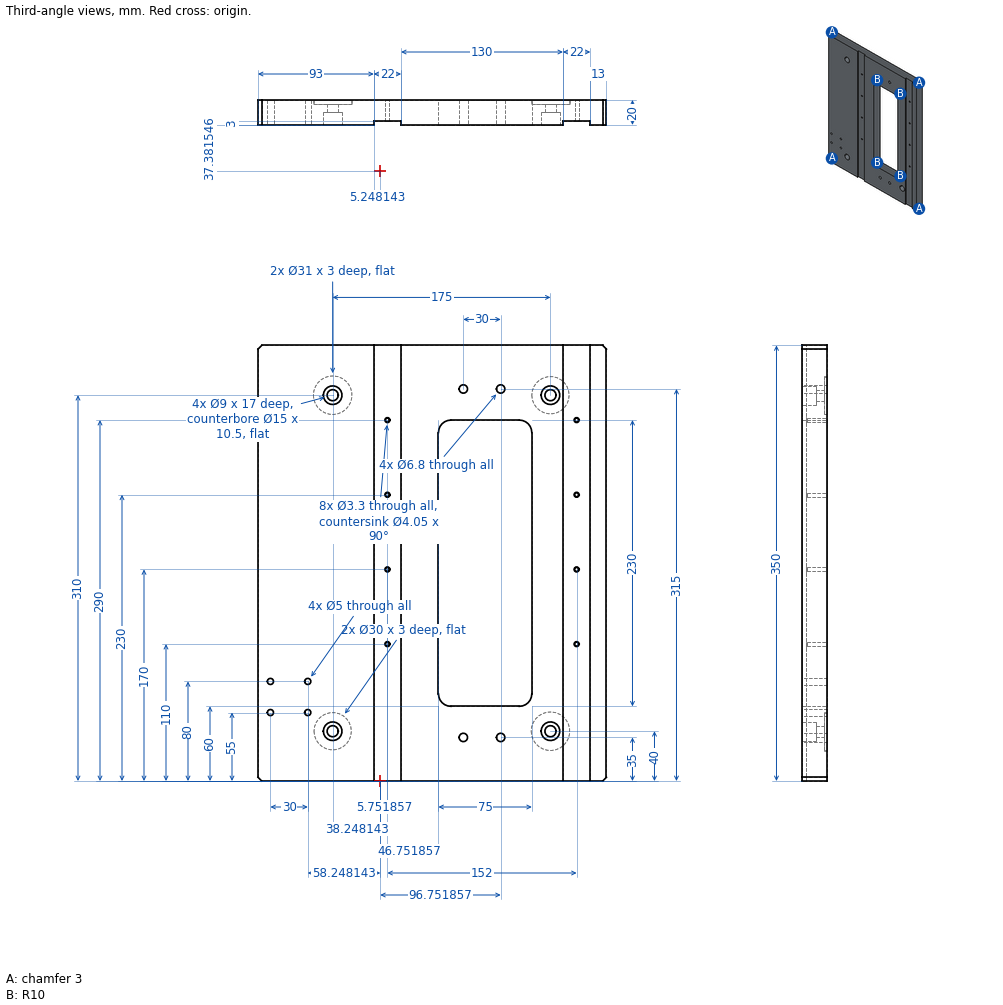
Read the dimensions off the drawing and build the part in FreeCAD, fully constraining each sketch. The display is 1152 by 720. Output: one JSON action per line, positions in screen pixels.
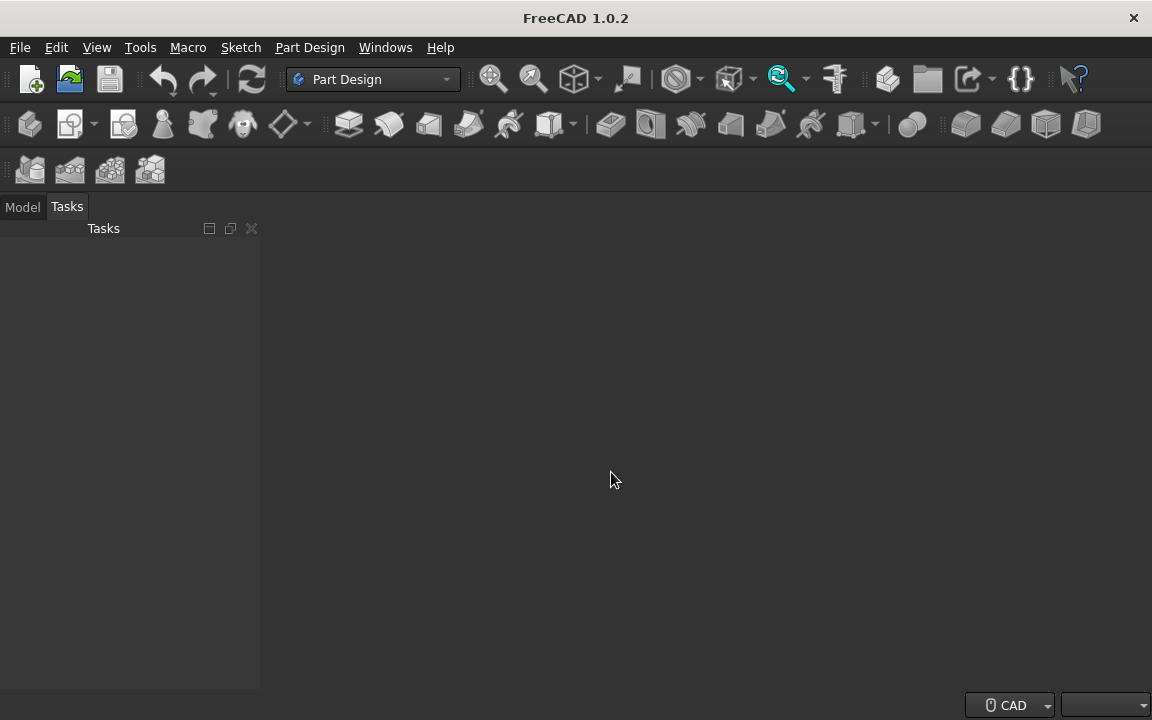
{"action": "left_click", "coordinate": [30, 80]}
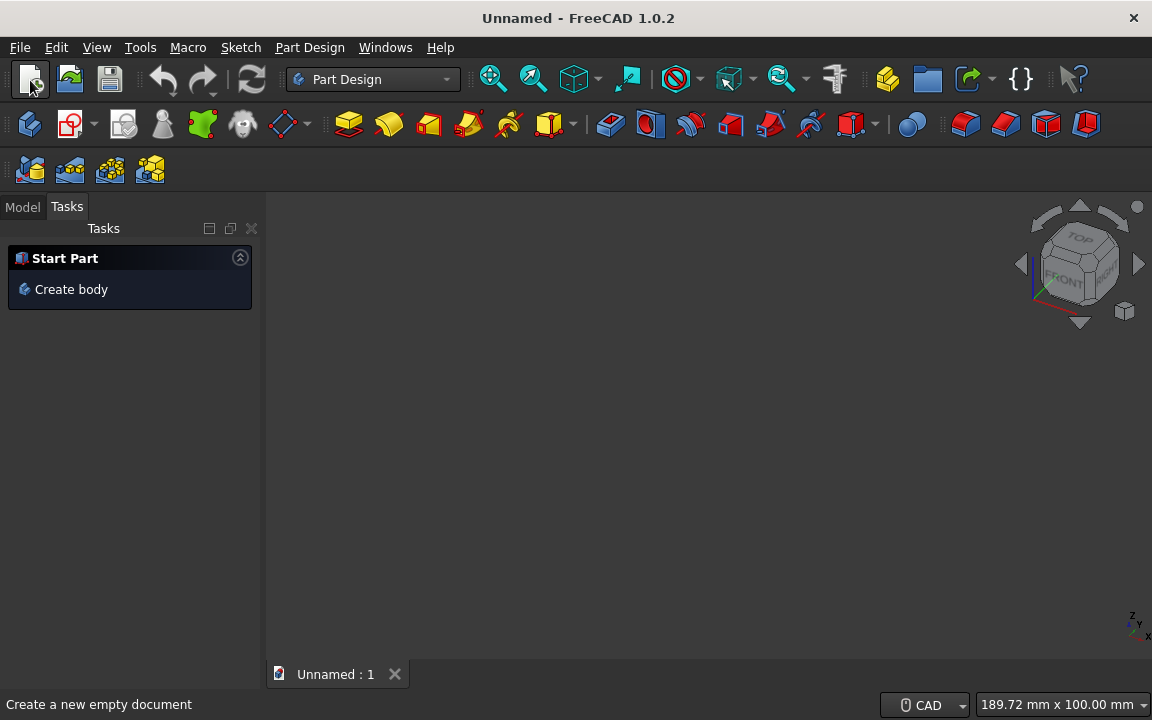
{"action": "left_click", "coordinate": [70, 124]}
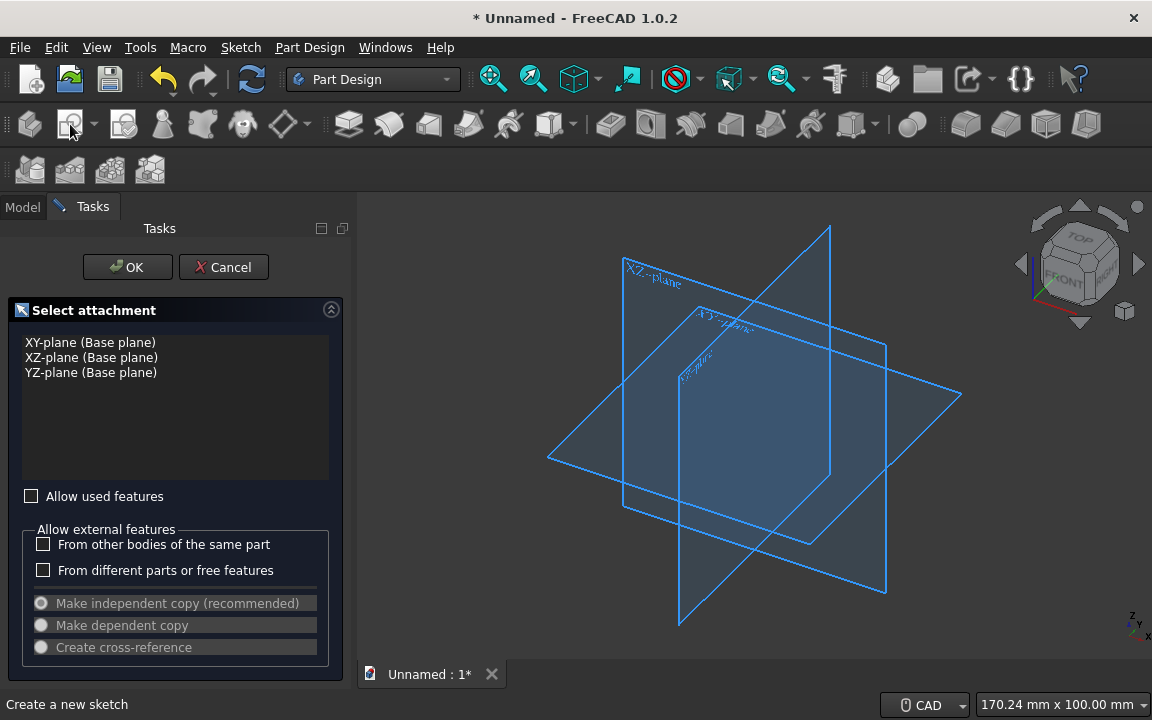
{"action": "left_click", "coordinate": [82, 342]}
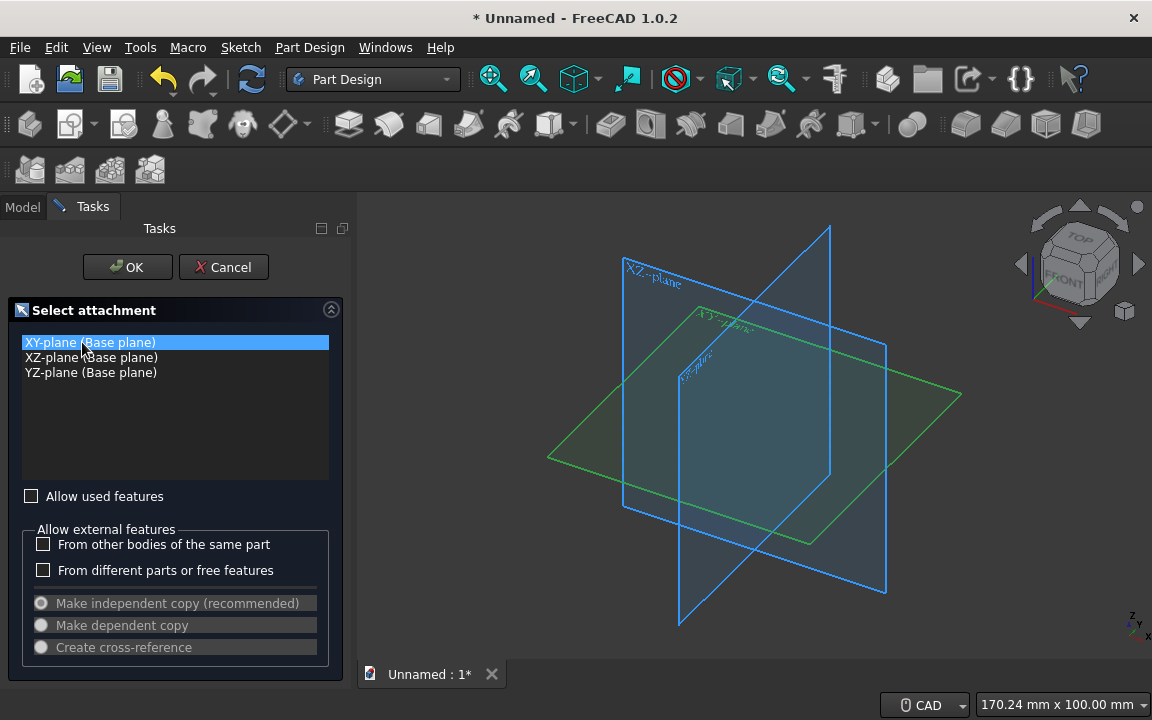
{"action": "left_click", "coordinate": [128, 267]}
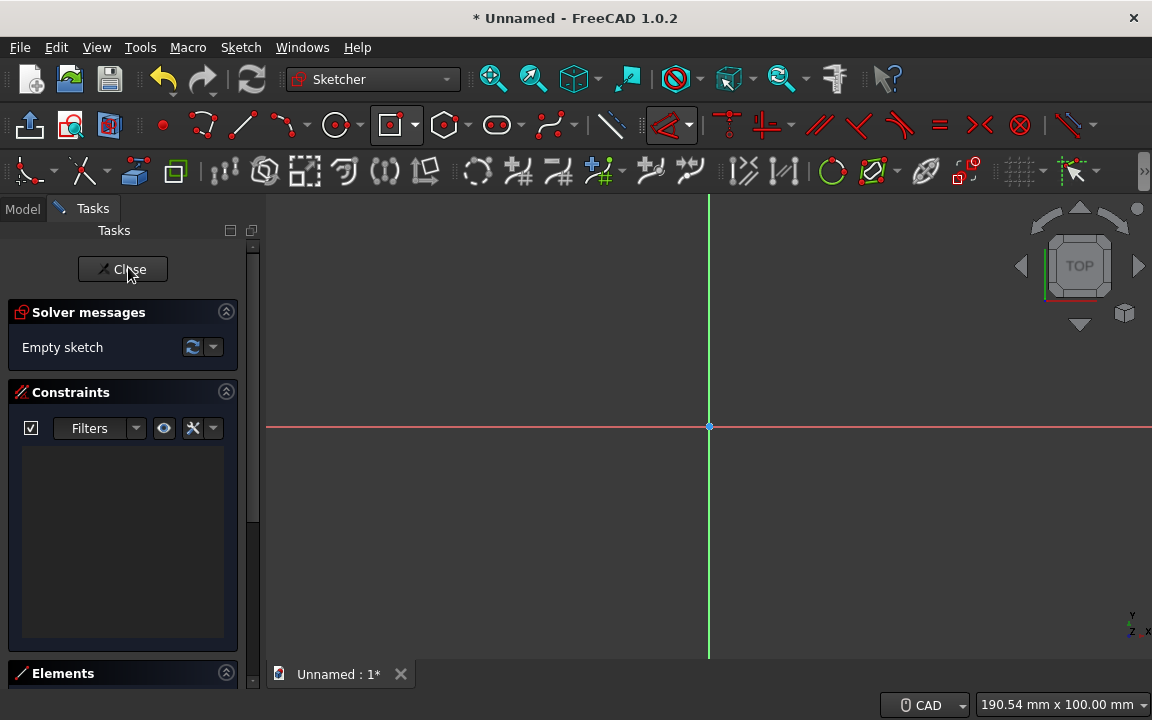
{"action": "scroll", "coordinate": [488, 504], "scroll_direction": "down", "scroll_amount": 5}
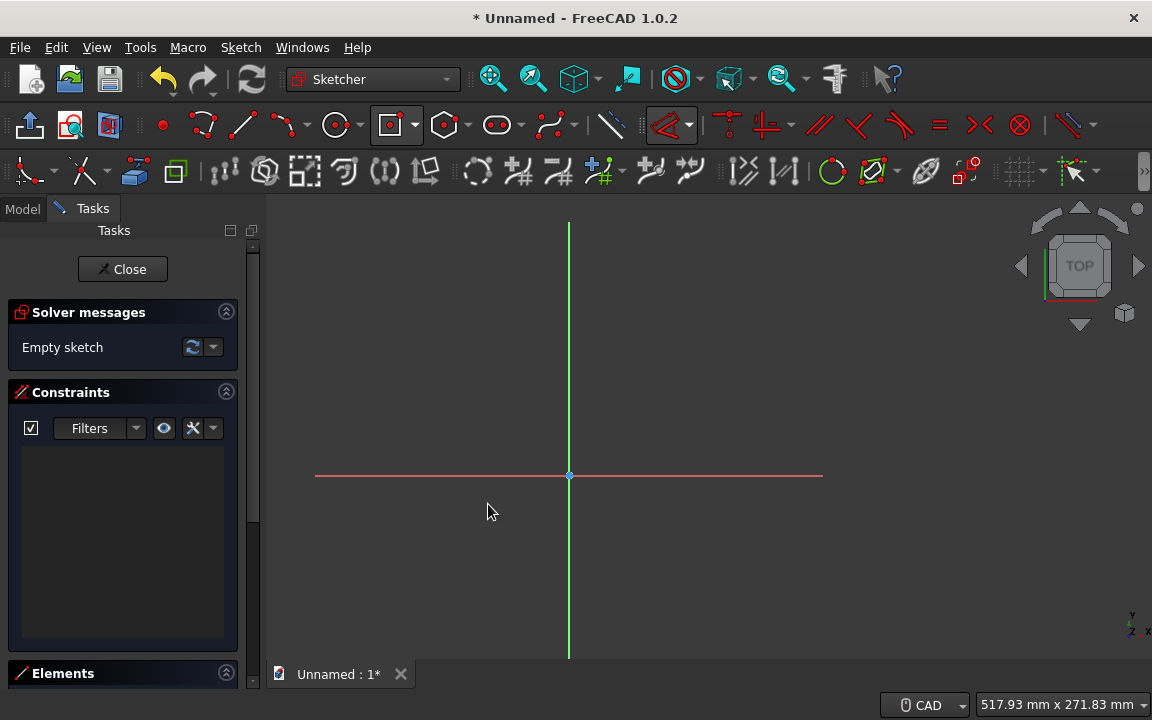
{"action": "left_click", "coordinate": [204, 126]}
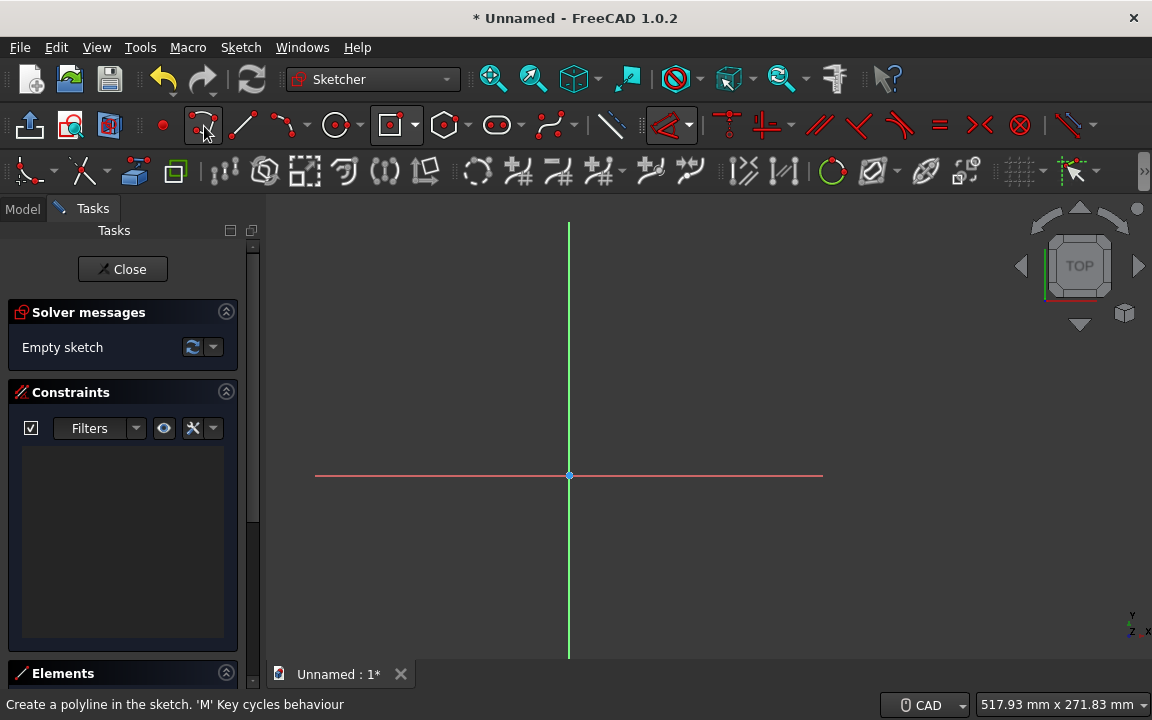
{"action": "scroll", "coordinate": [560, 412], "scroll_direction": "up", "scroll_amount": 3}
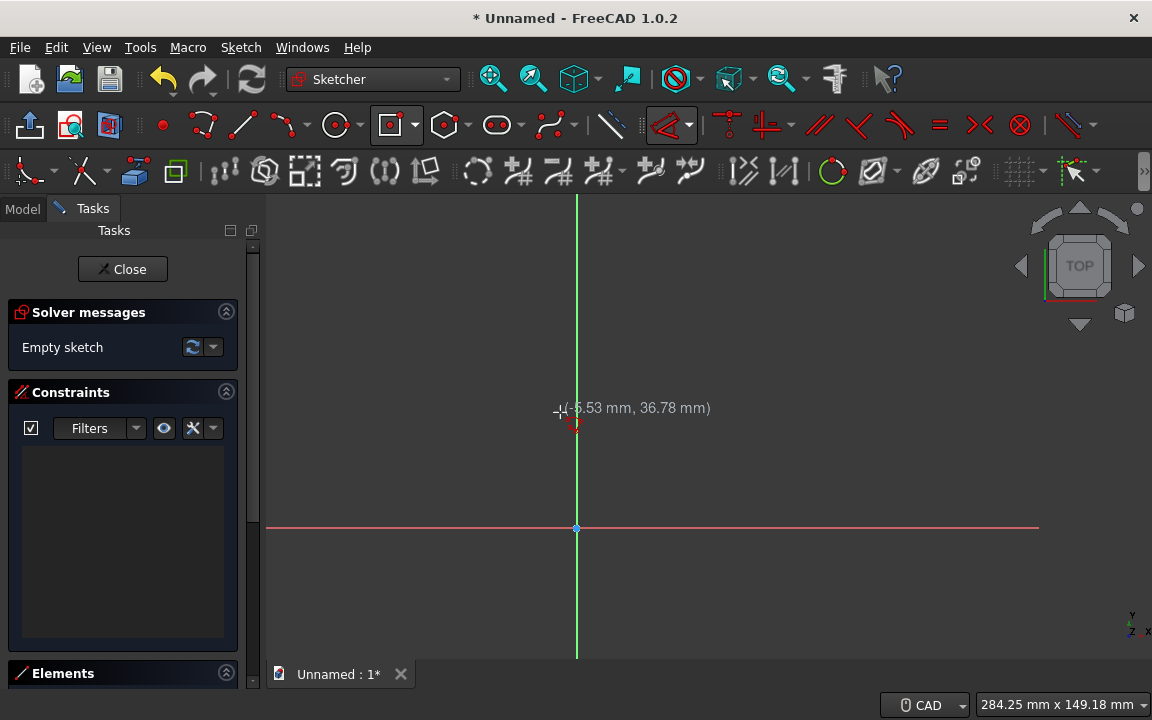
{"action": "left_click", "coordinate": [561, 412]}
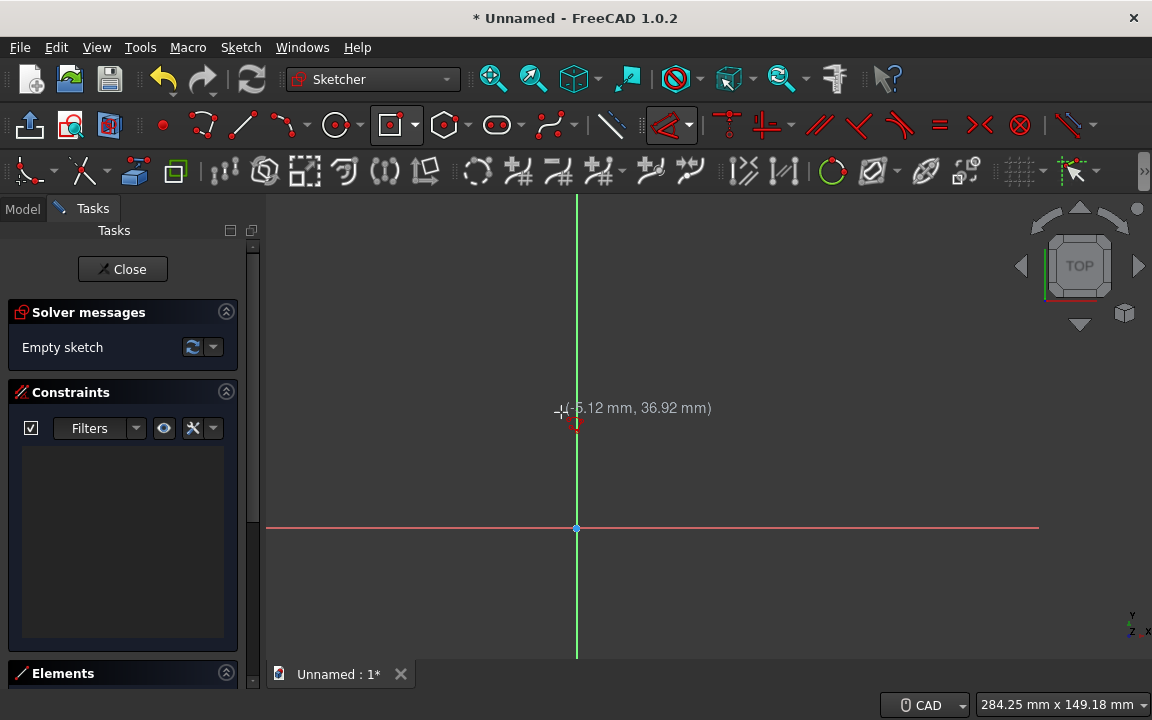
{"action": "scroll", "coordinate": [561, 402], "scroll_direction": "up", "scroll_amount": 3}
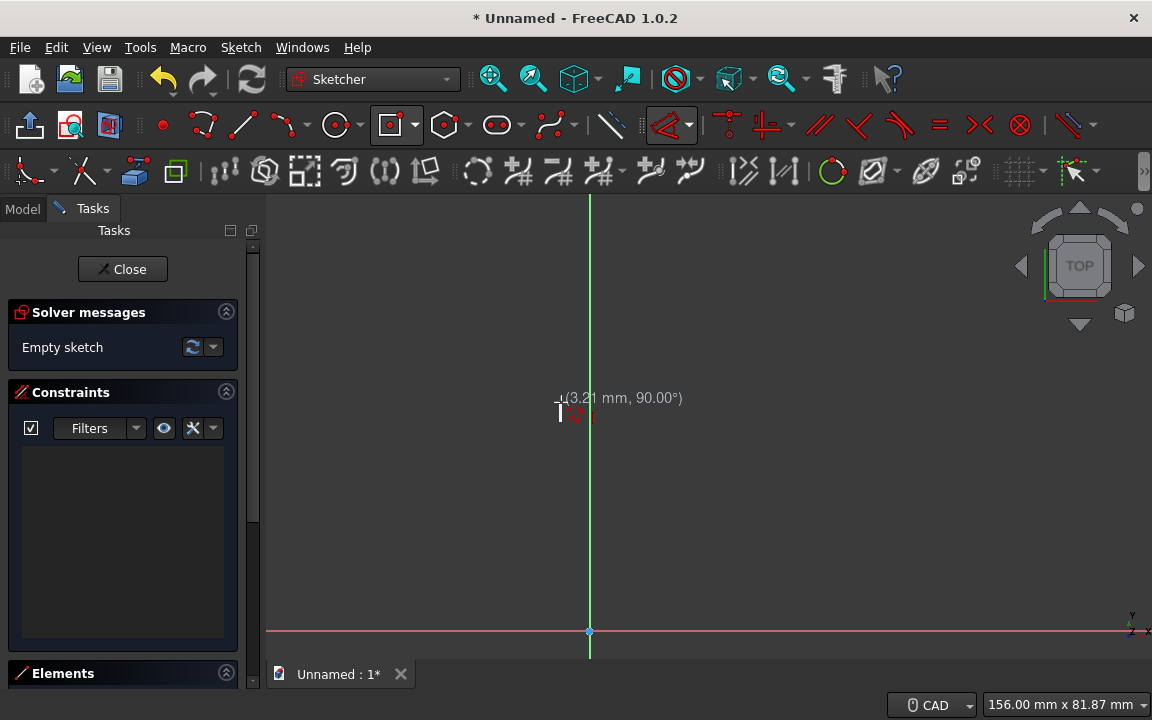
{"action": "left_click", "coordinate": [561, 402]}
{"action": "left_click", "coordinate": [685, 402]}
{"action": "left_click", "coordinate": [685, 419]}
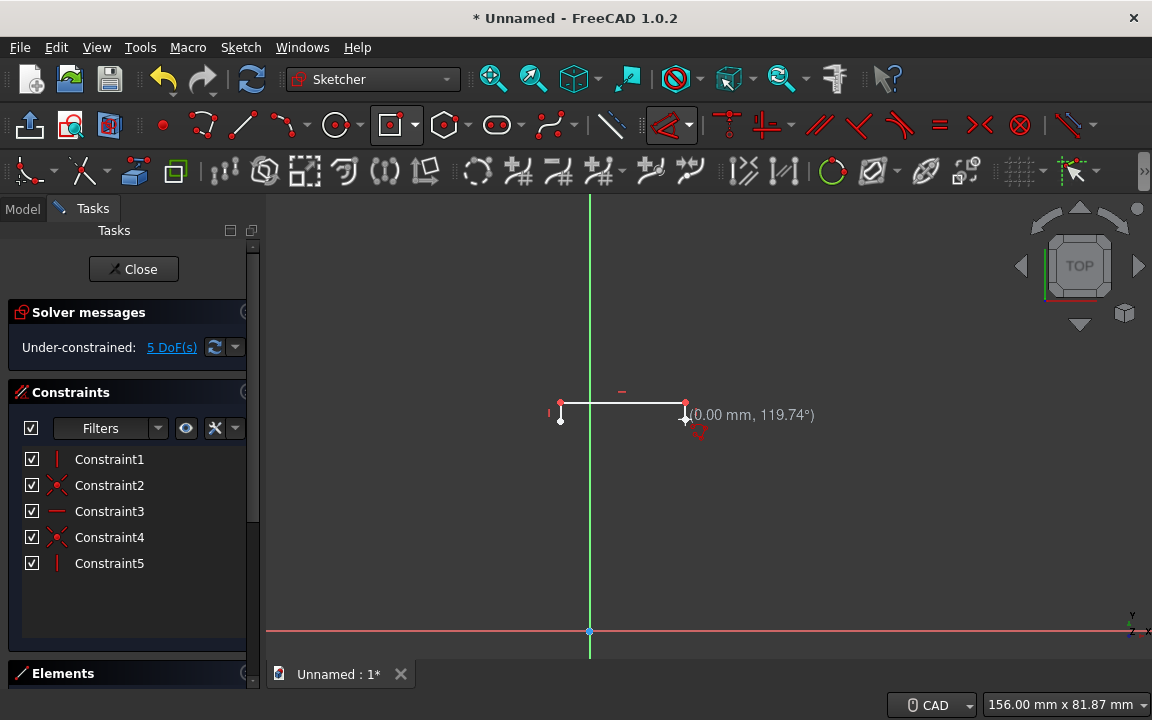
{"action": "scroll", "coordinate": [560, 408], "scroll_direction": "down", "scroll_amount": 6}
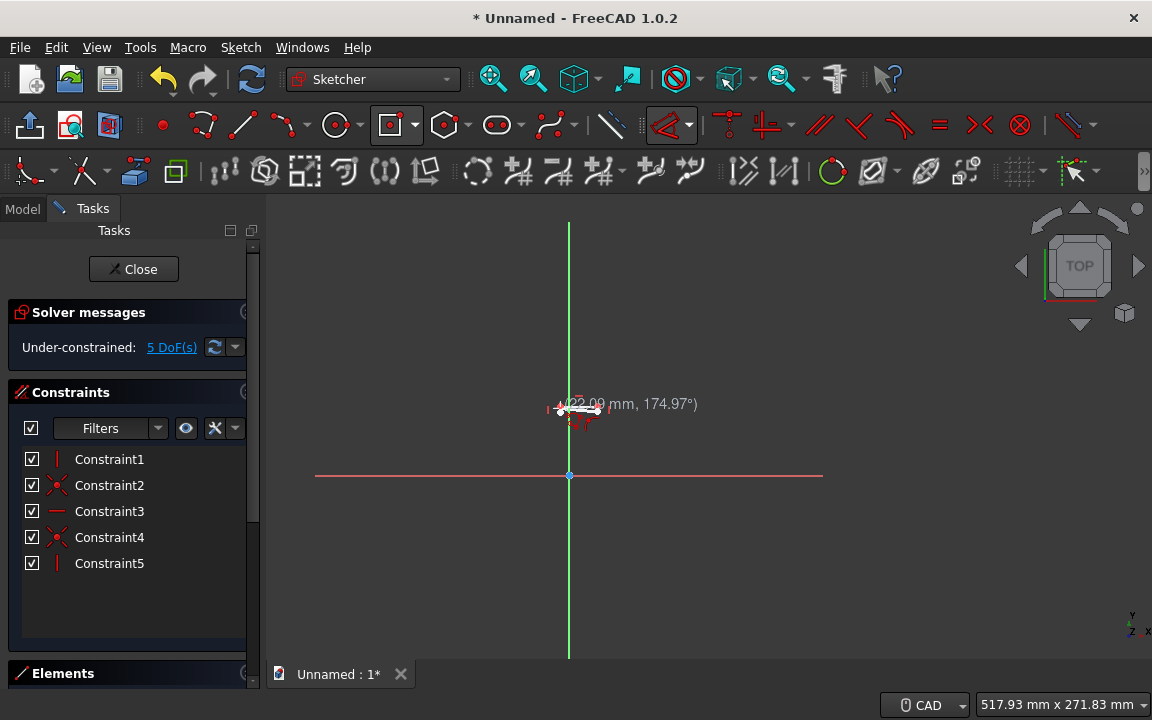
{"action": "left_click", "coordinate": [820, 412]}